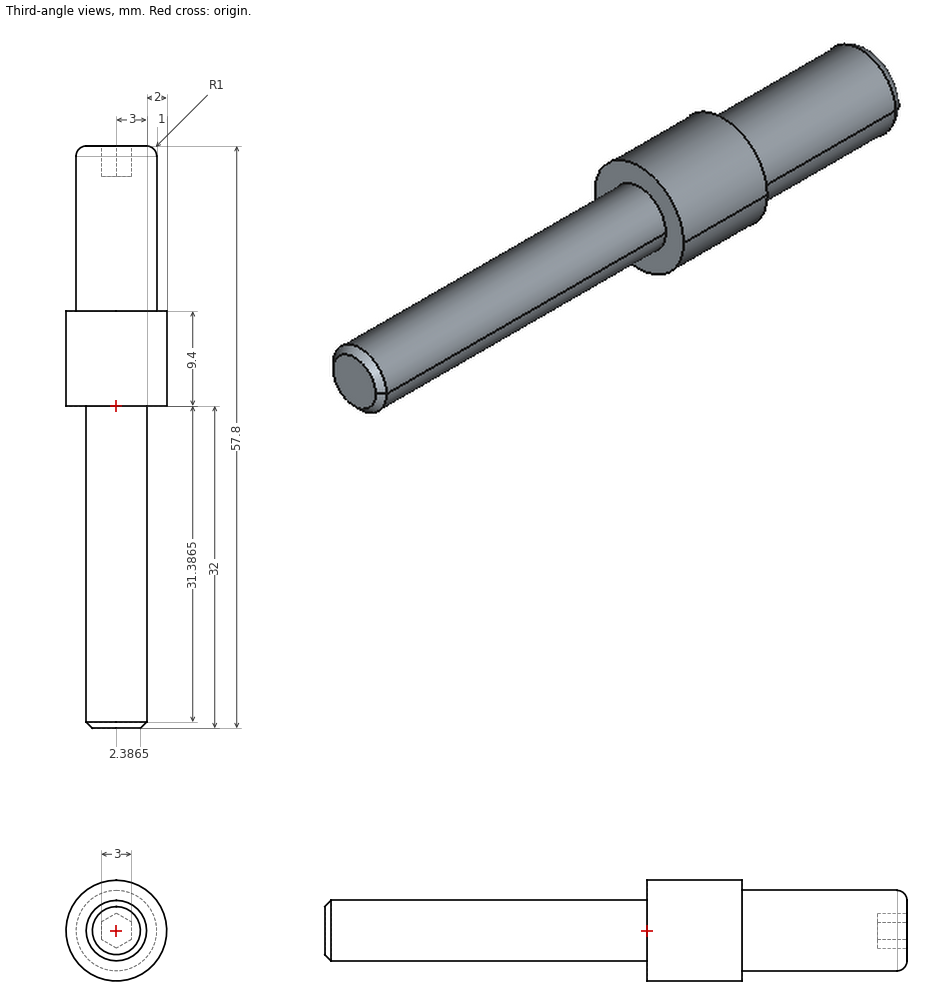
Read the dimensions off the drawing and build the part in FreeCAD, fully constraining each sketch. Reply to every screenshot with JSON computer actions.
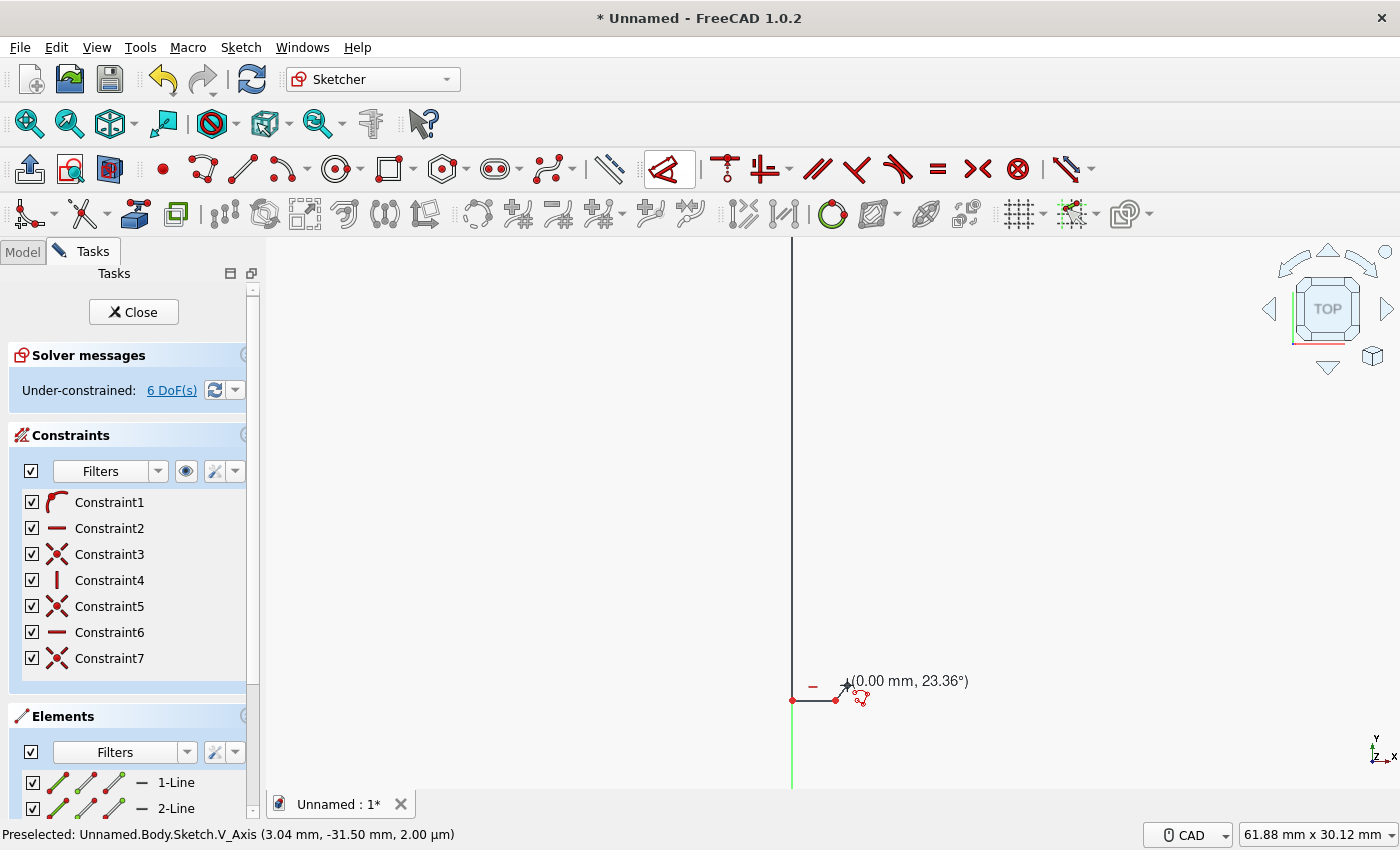
{"action": "scroll", "coordinate": [733, 662], "scroll_direction": "down", "scroll_amount": 6}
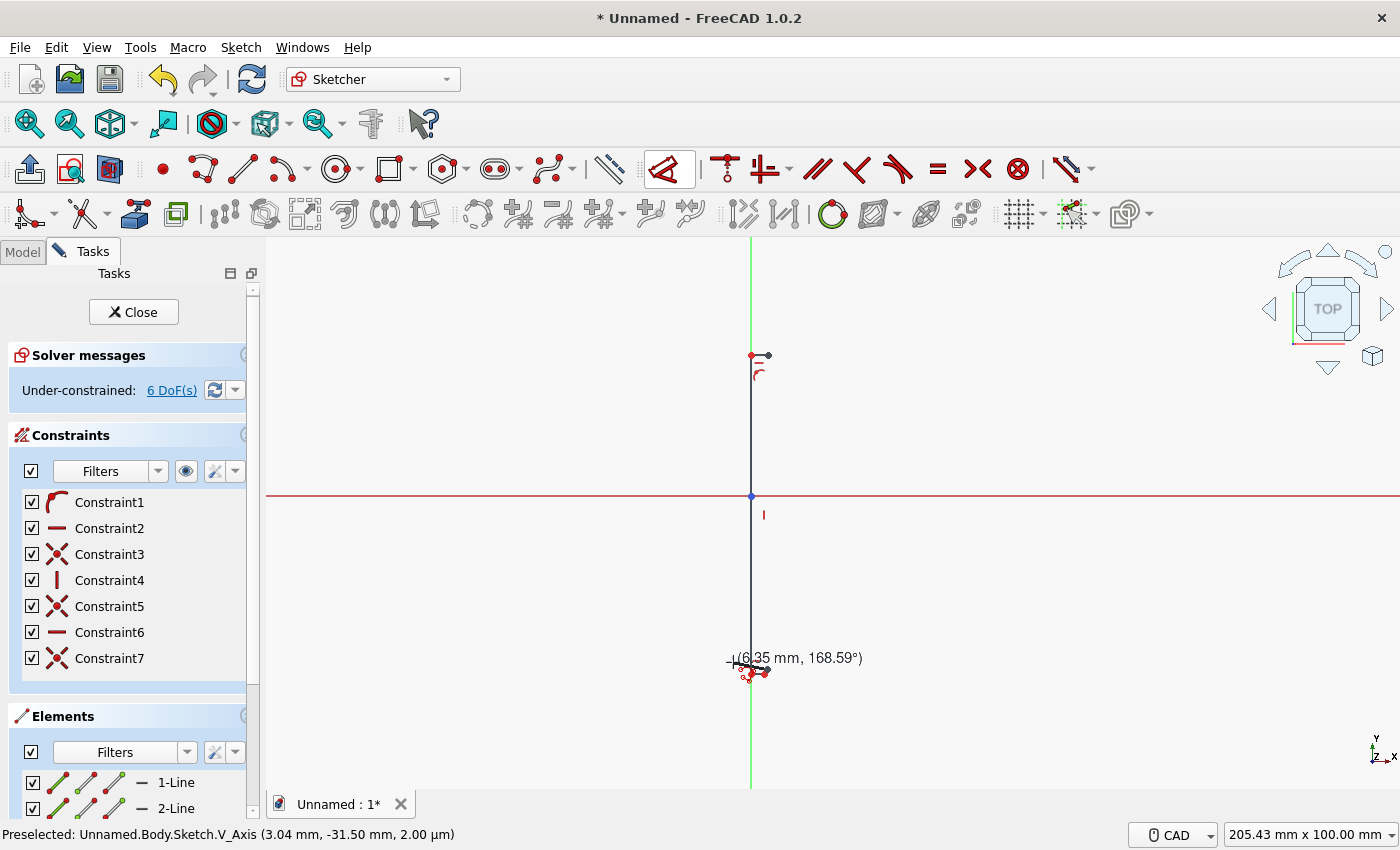
{"action": "left_click", "coordinate": [768, 496]}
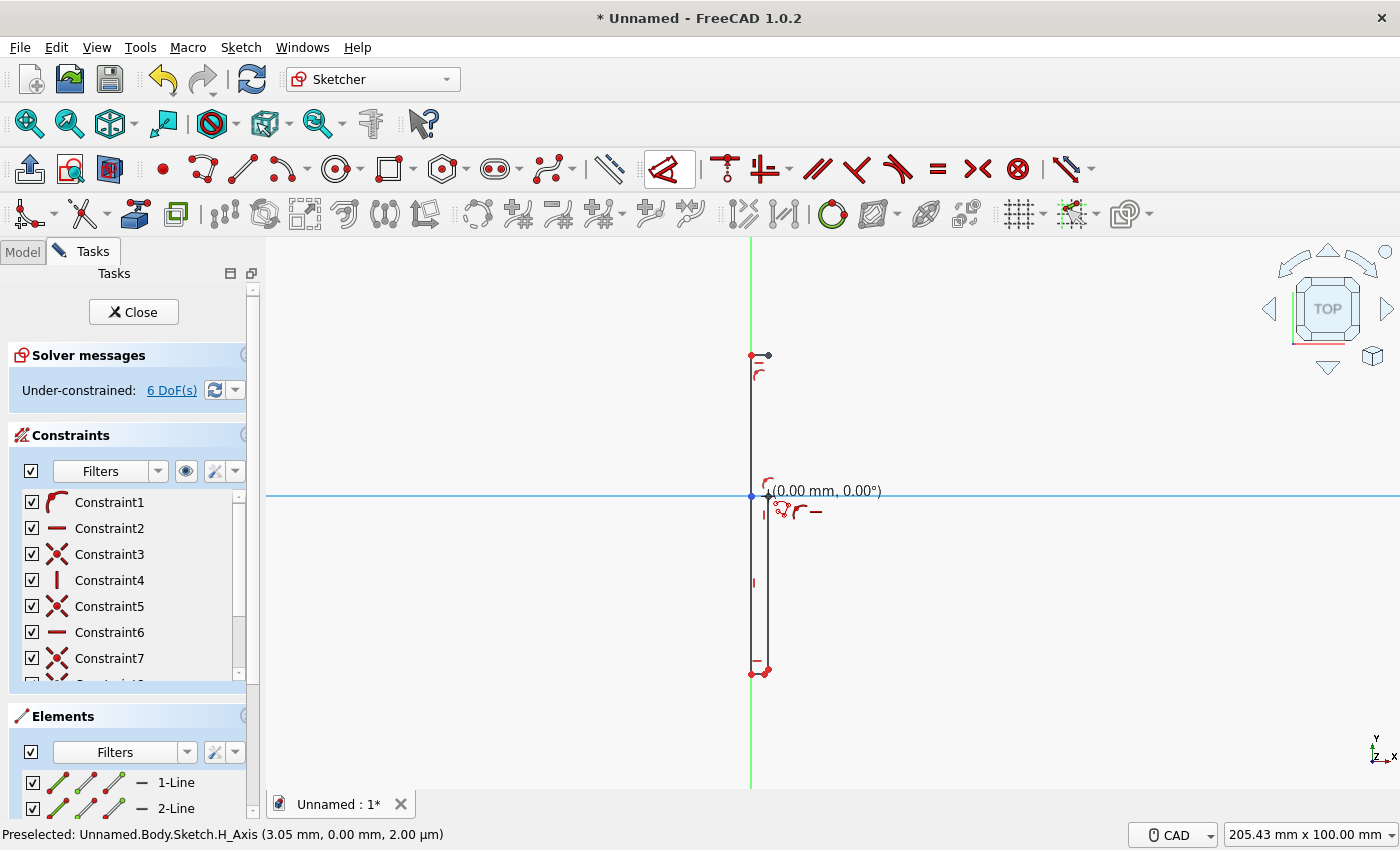
{"action": "scroll", "coordinate": [779, 496], "scroll_direction": "up", "scroll_amount": 2}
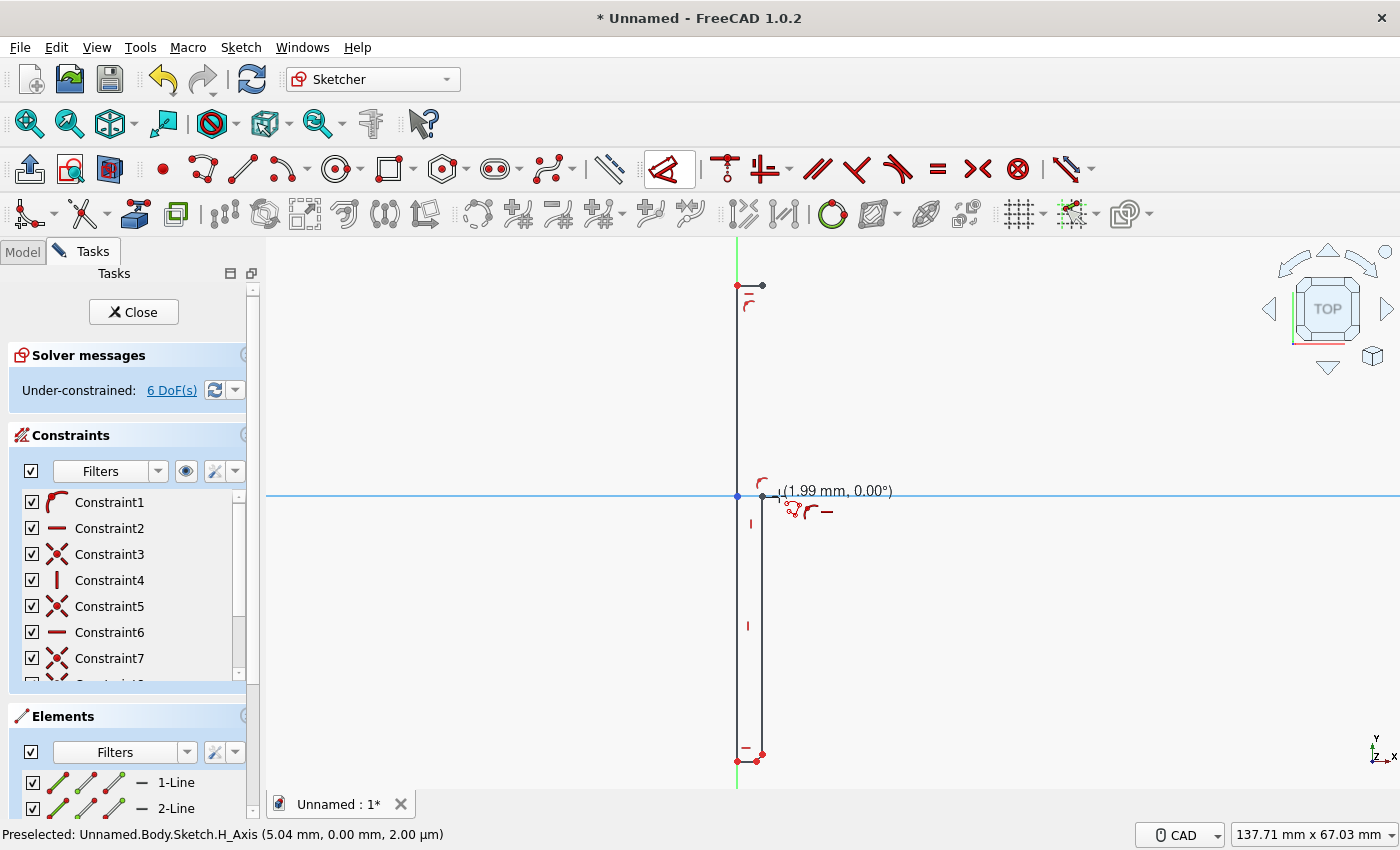
{"action": "left_click", "coordinate": [778, 505]}
{"action": "left_click", "coordinate": [778, 419]}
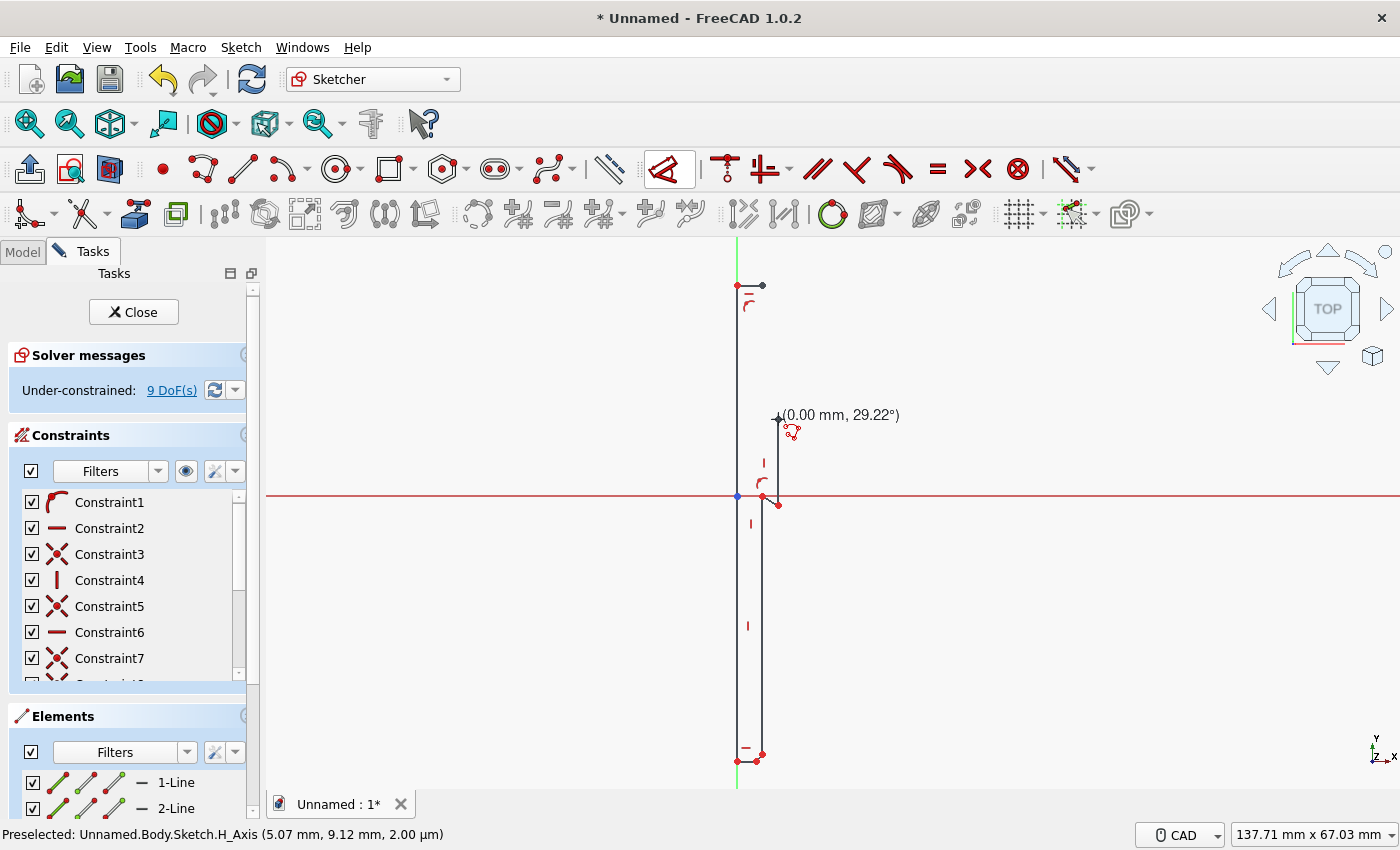
{"action": "scroll", "coordinate": [770, 419], "scroll_direction": "up", "scroll_amount": 4}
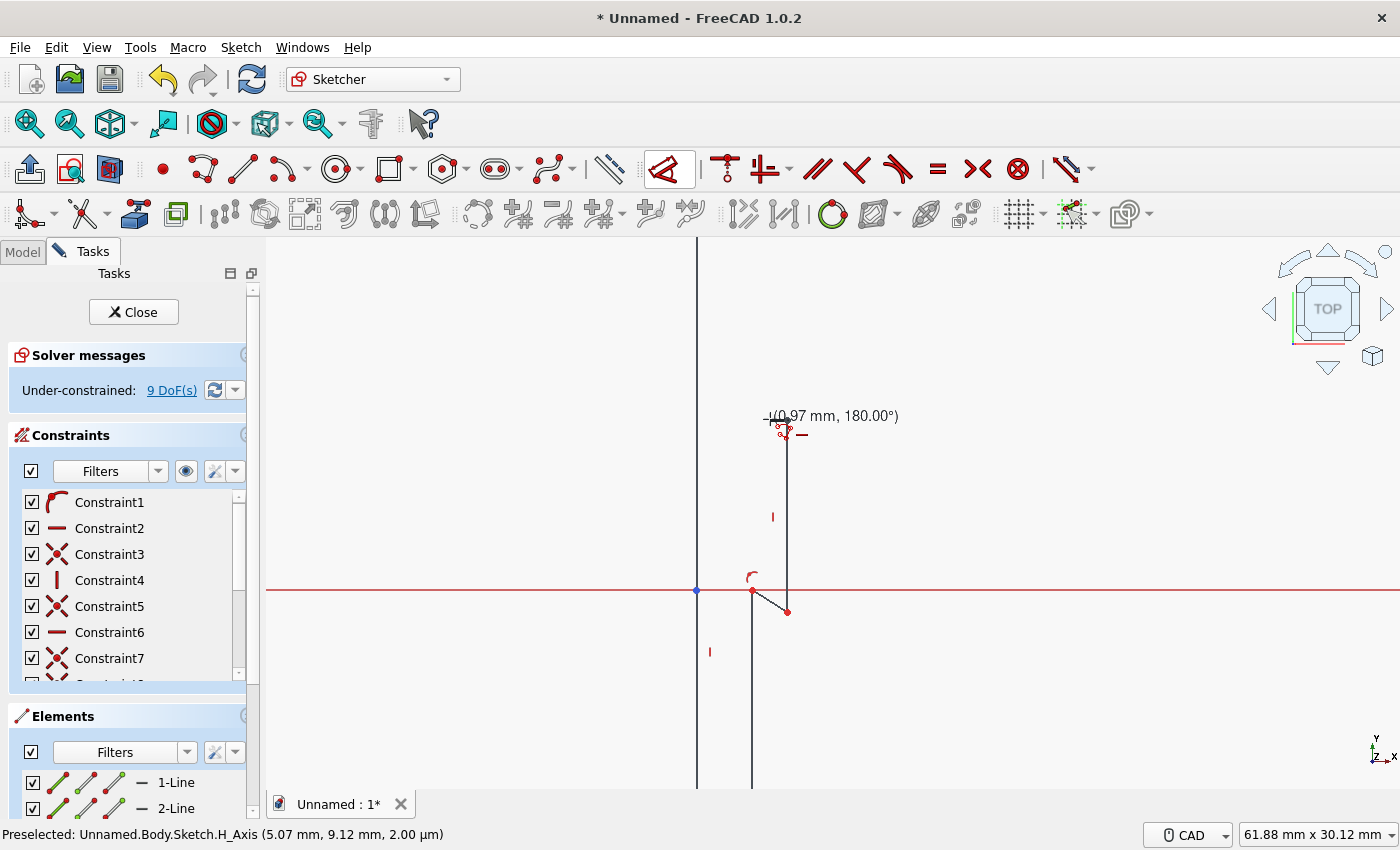
{"action": "left_click", "coordinate": [770, 419]}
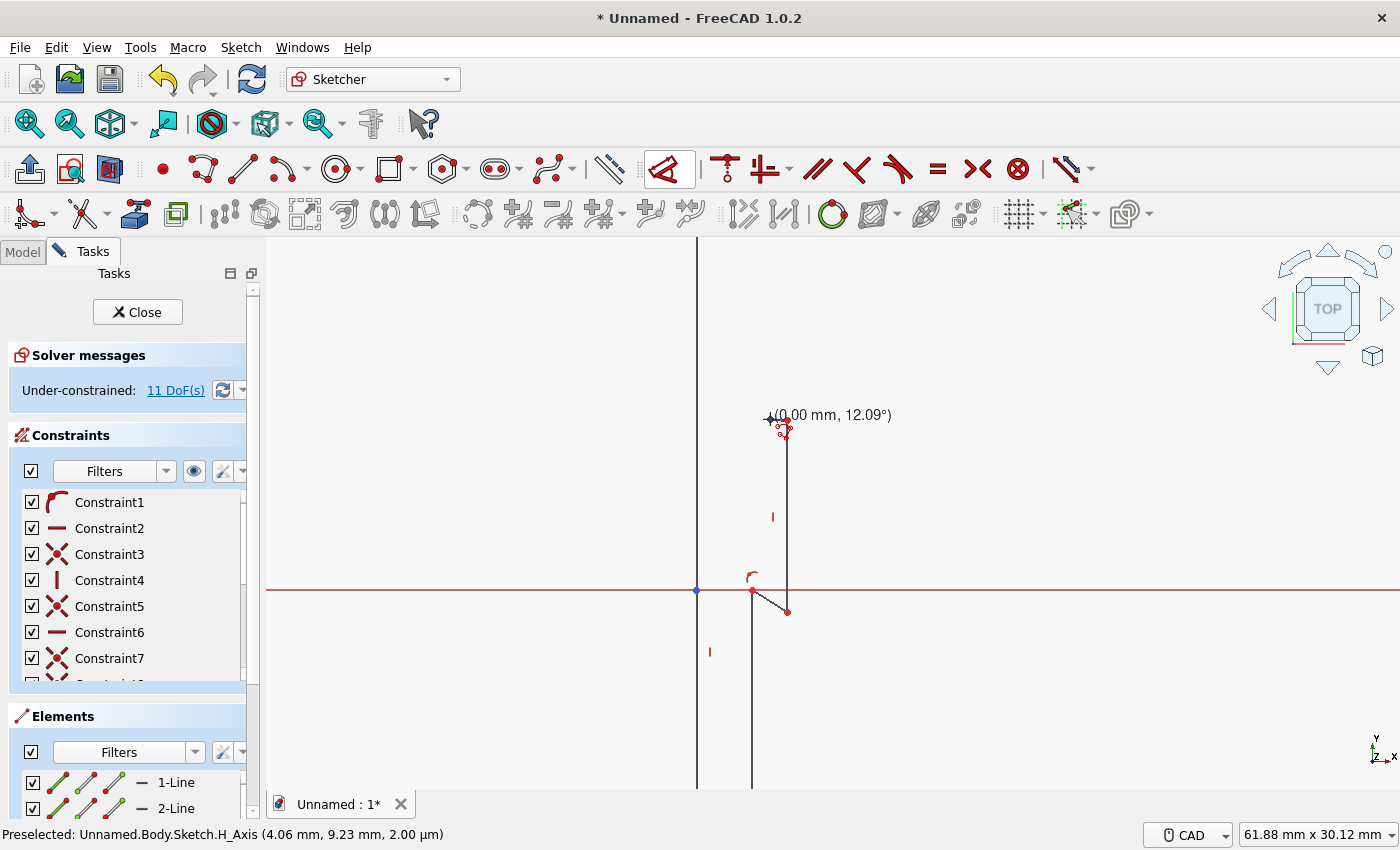
{"action": "scroll", "coordinate": [774, 455], "scroll_direction": "down", "scroll_amount": 6}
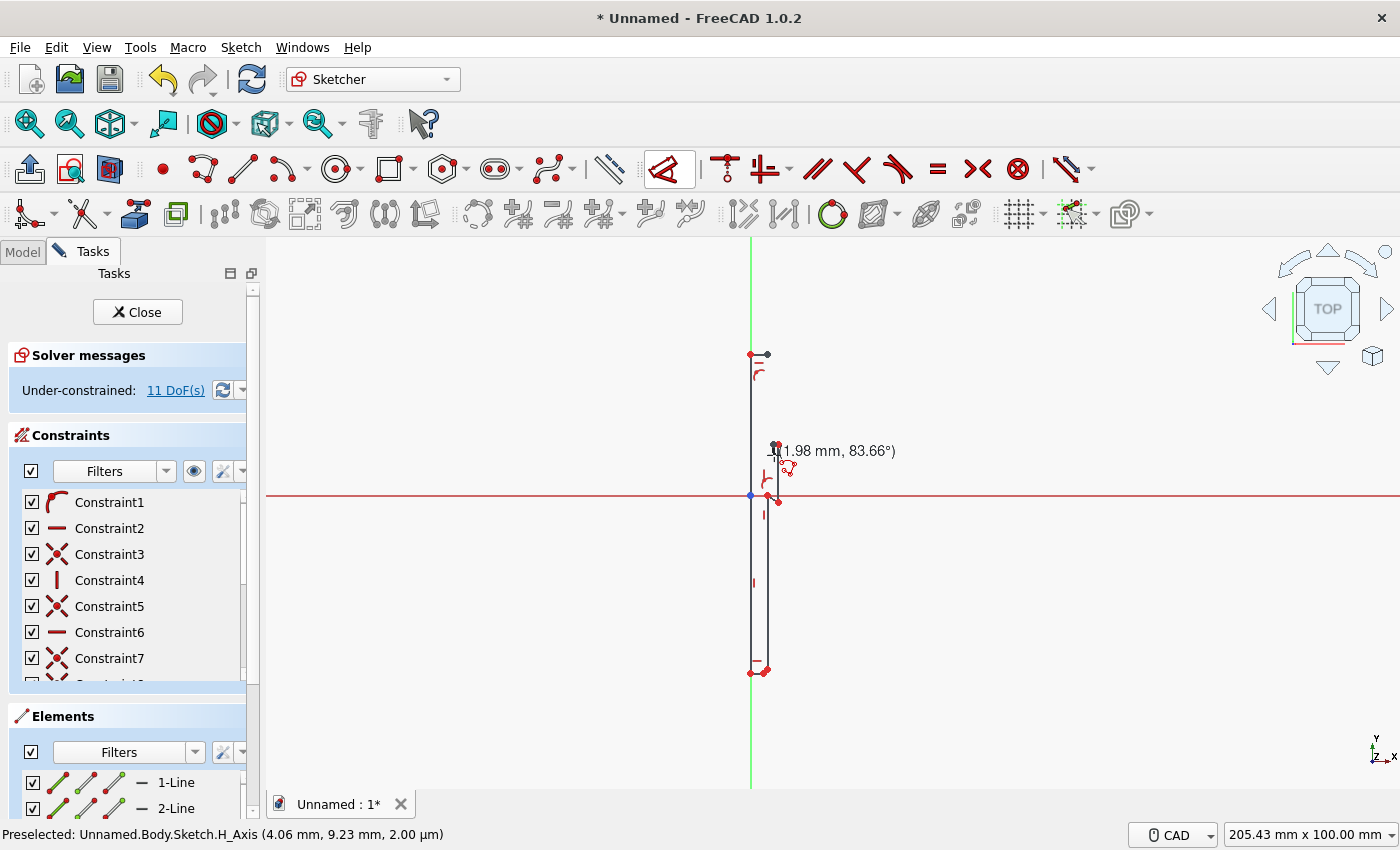
{"action": "scroll", "coordinate": [773, 359], "scroll_direction": "up", "scroll_amount": 4}